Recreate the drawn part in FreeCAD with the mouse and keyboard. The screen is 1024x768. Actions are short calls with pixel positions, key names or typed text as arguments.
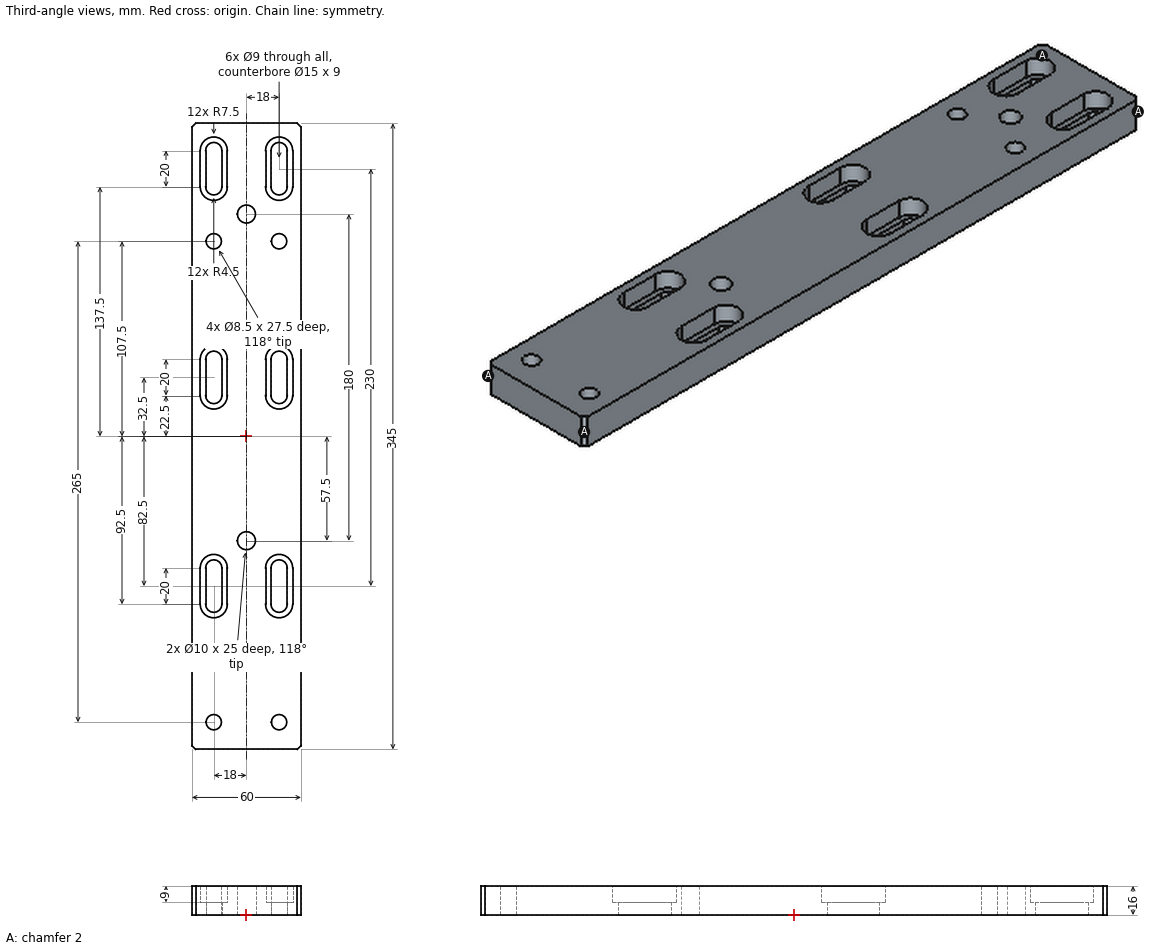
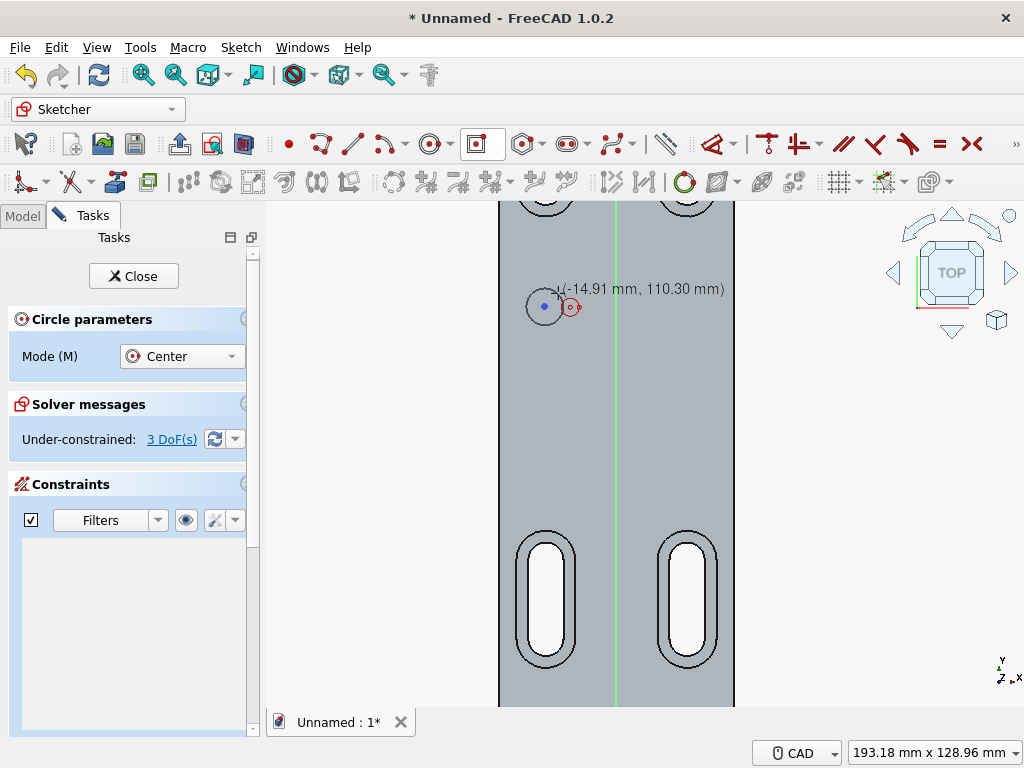
scroll(687, 305, up, 2)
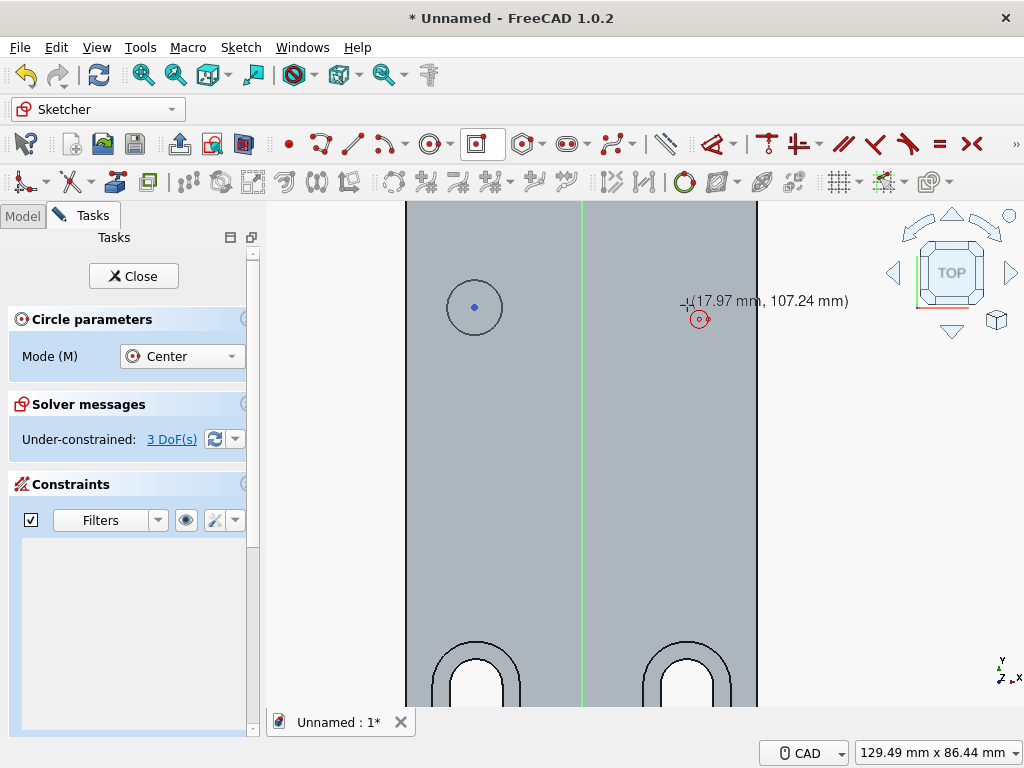
scroll(575, 296, down, 8)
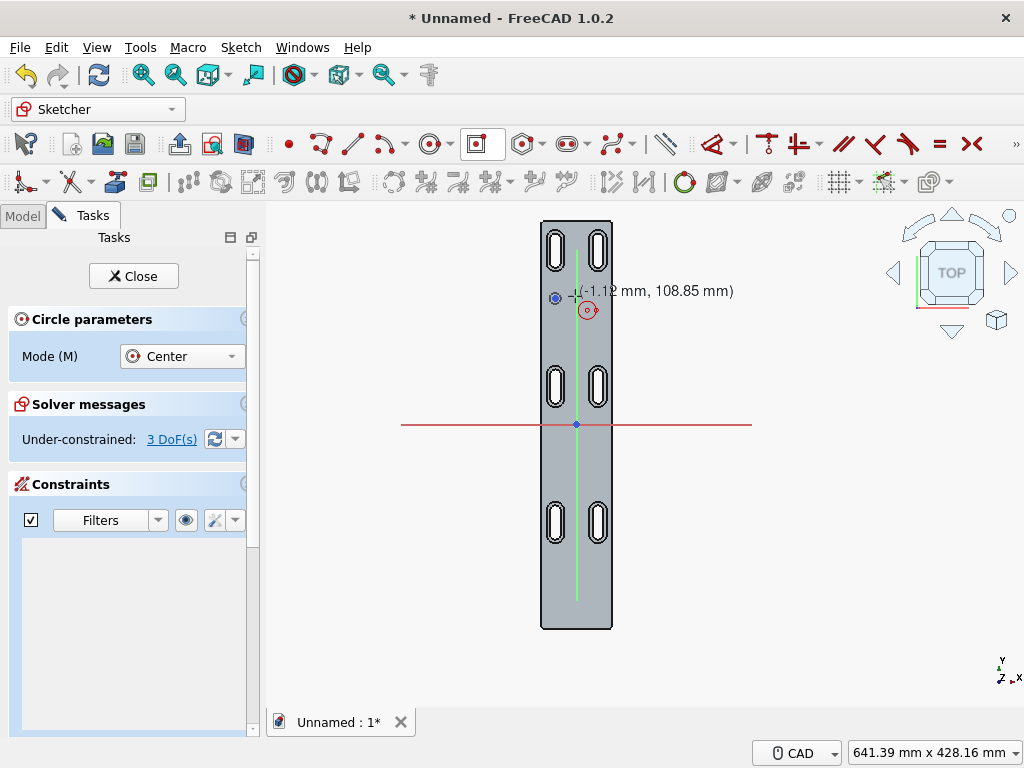
click(598, 298)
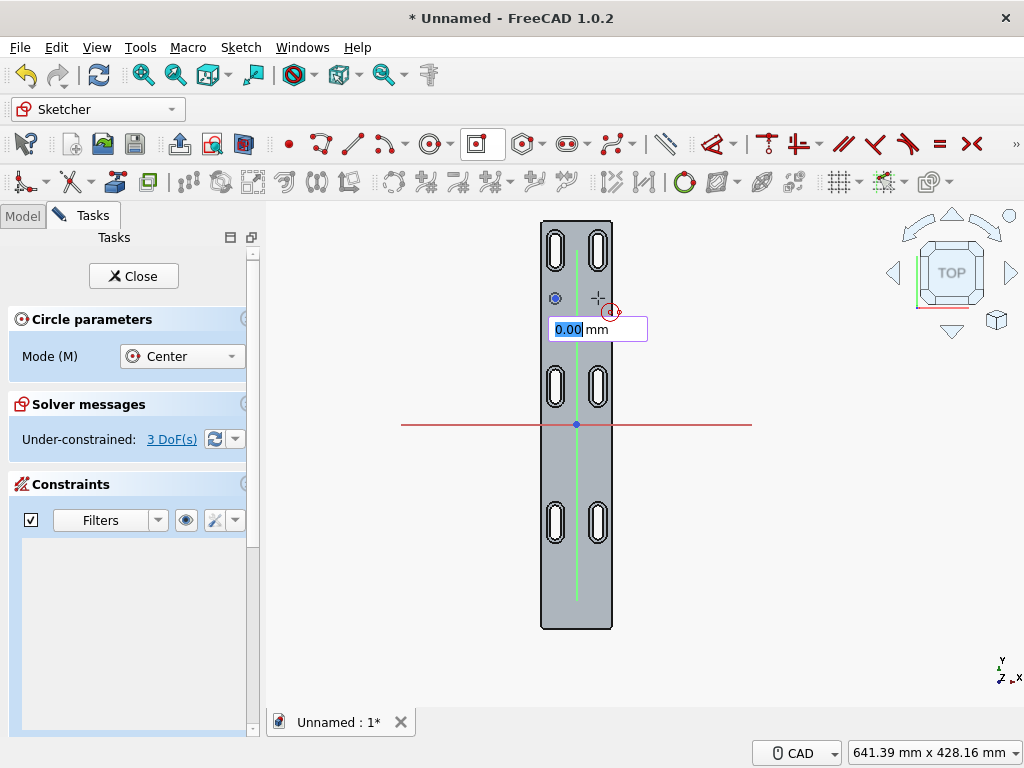
scroll(601, 294, up, 6)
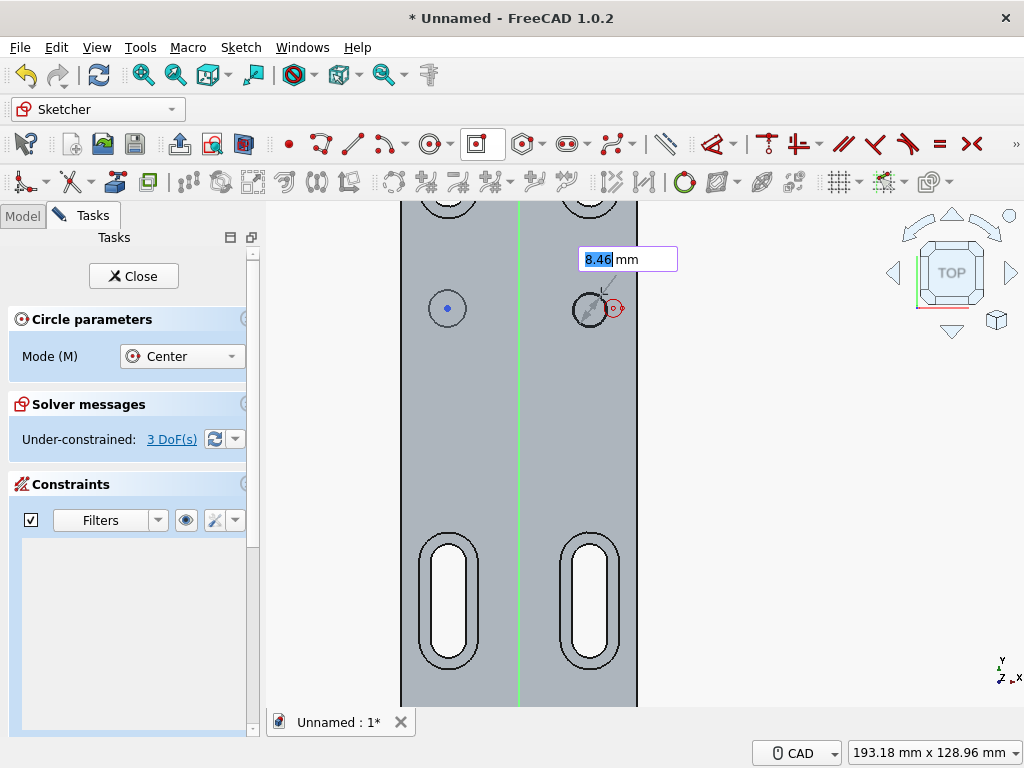
click(602, 295)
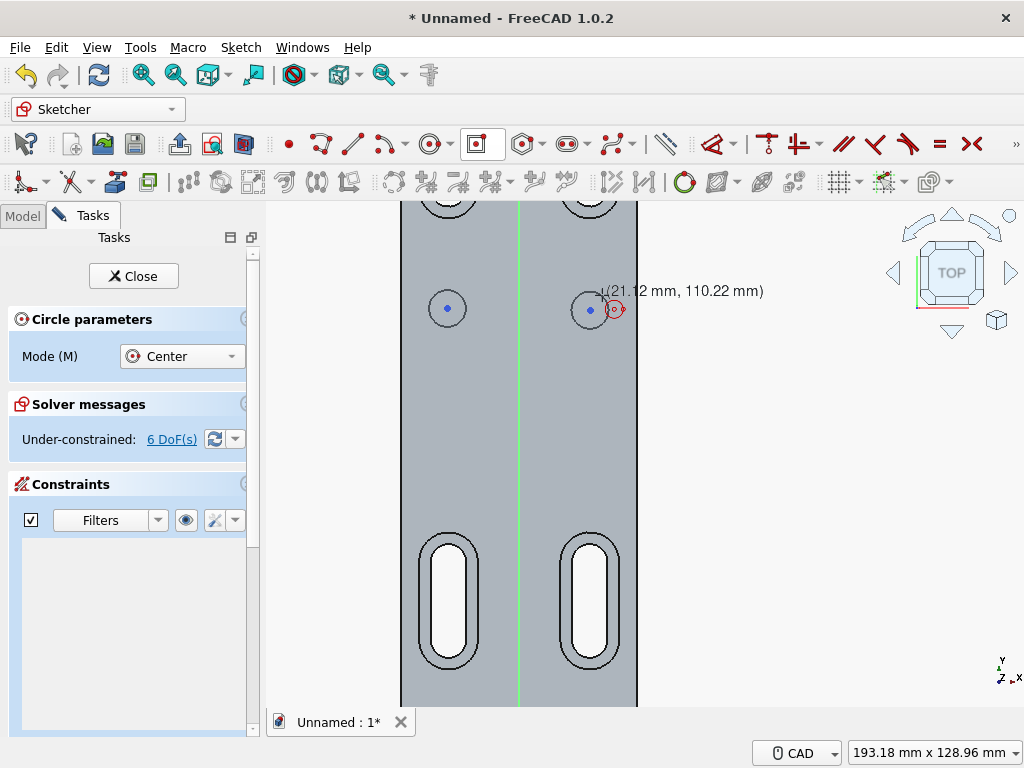
scroll(601, 293, down, 6)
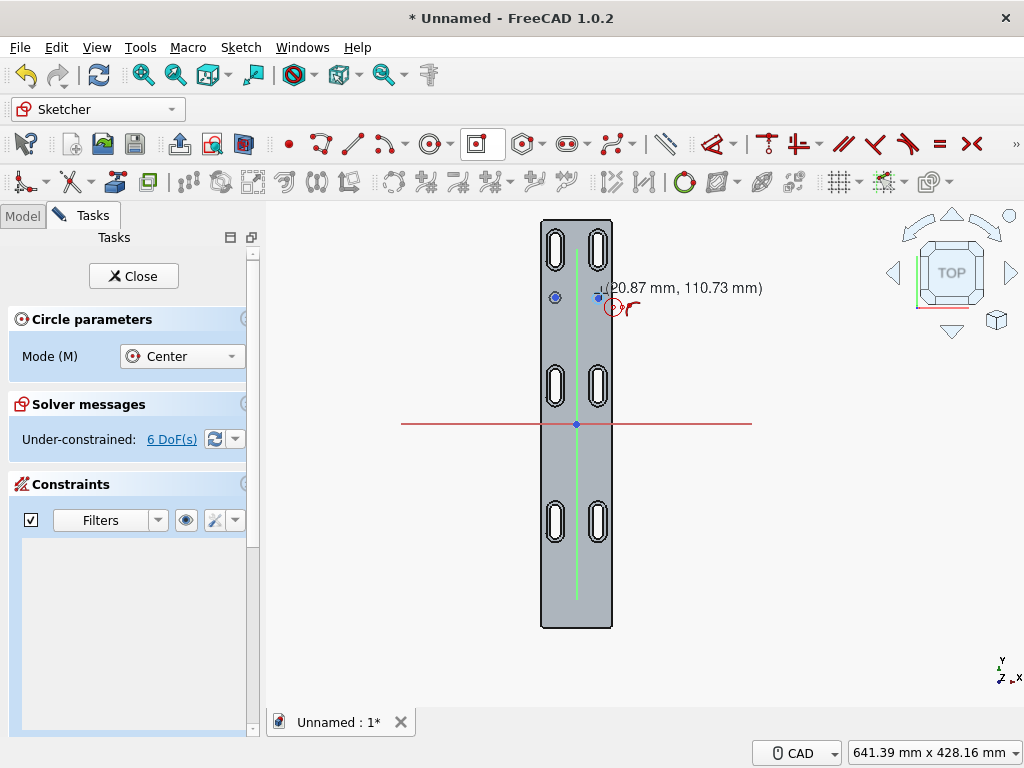
scroll(555, 610, up, 8)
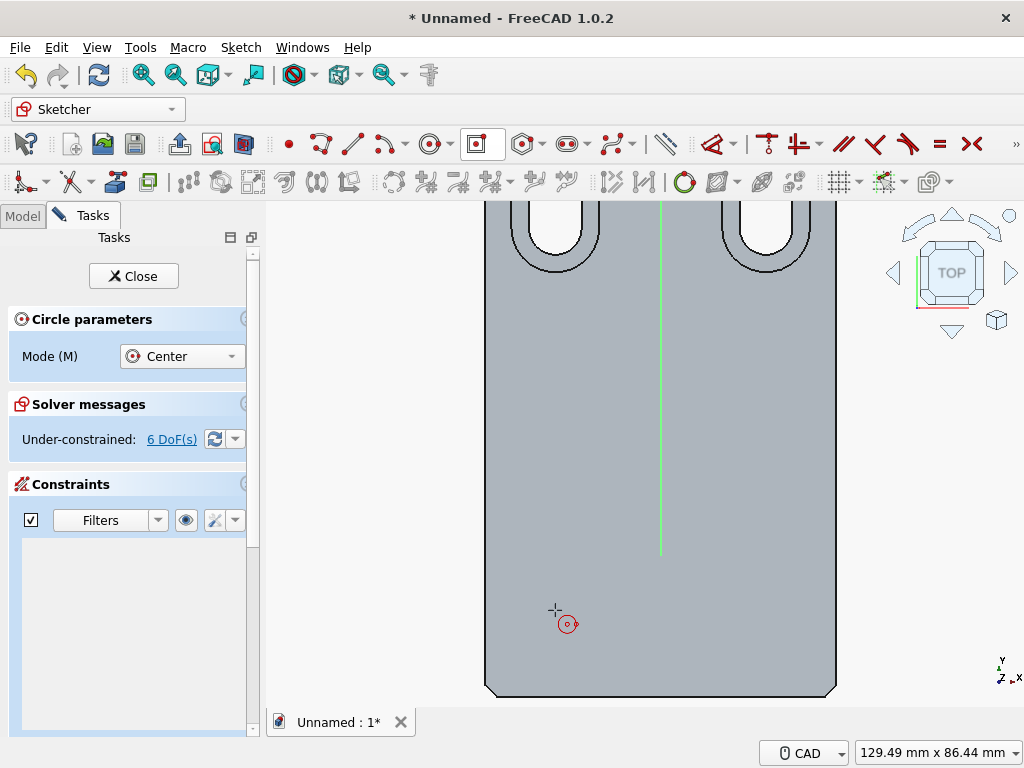
scroll(555, 611, down, 8)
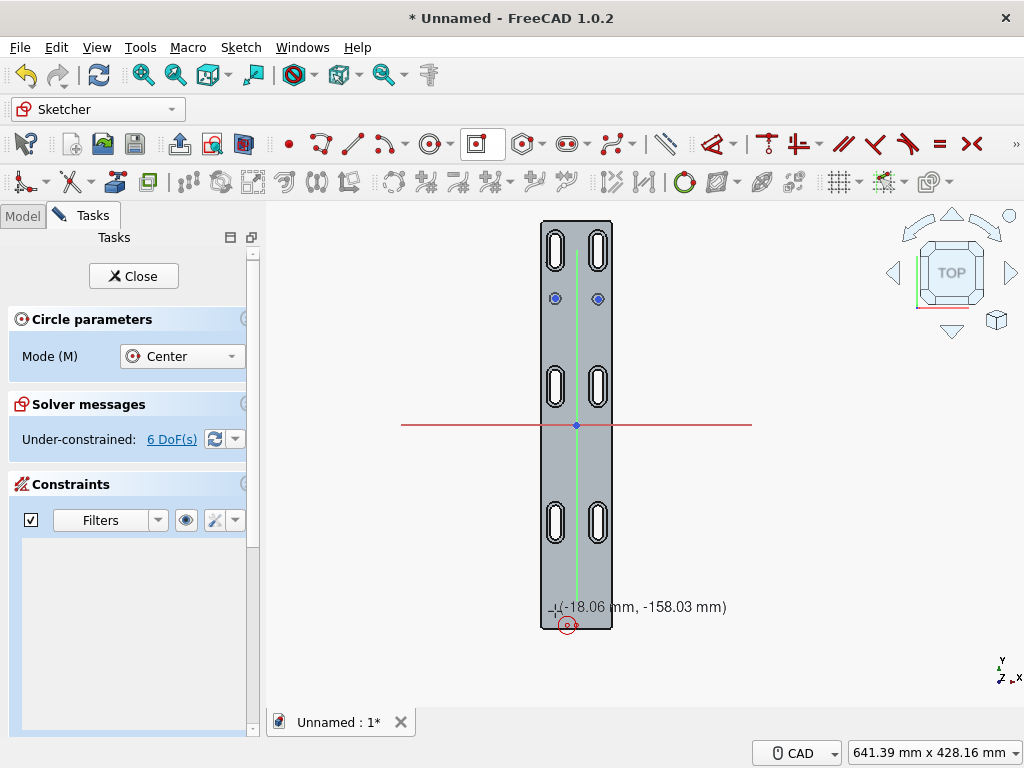
click(555, 611)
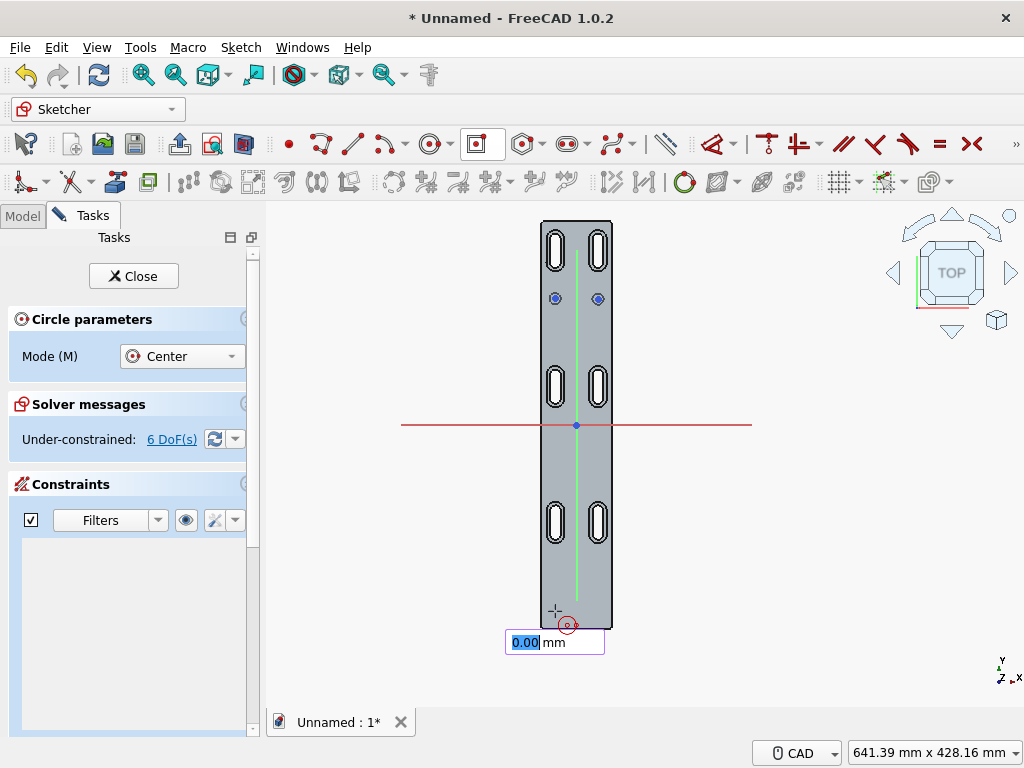
scroll(559, 608, up, 6)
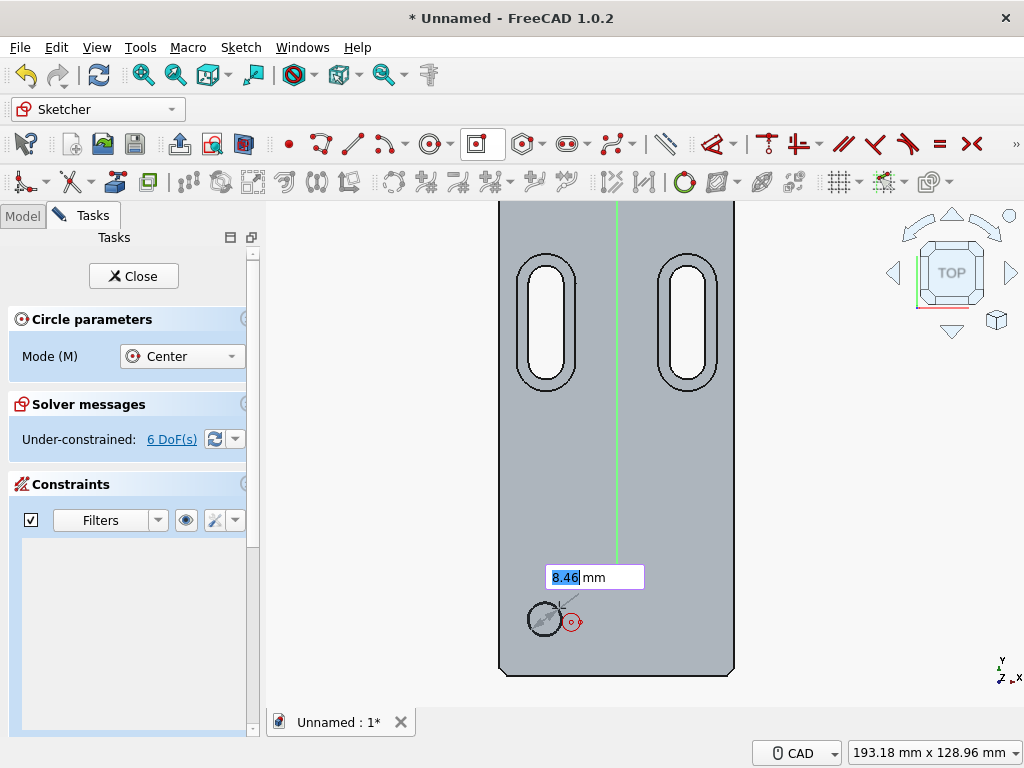
click(558, 605)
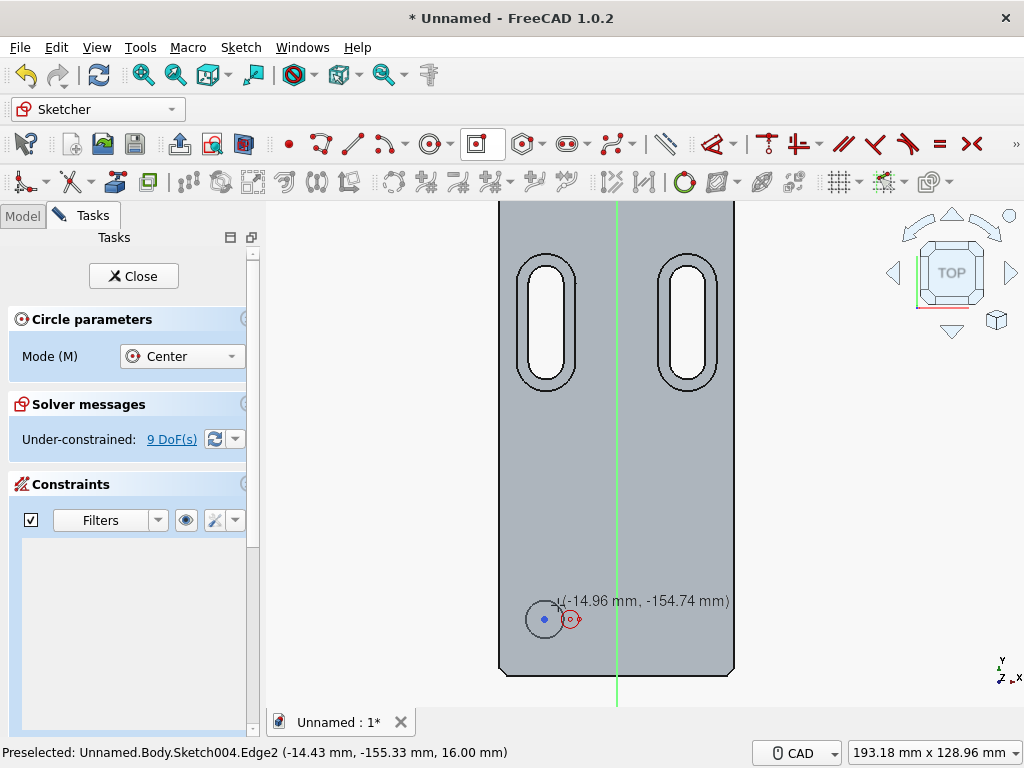
scroll(687, 617, up, 2)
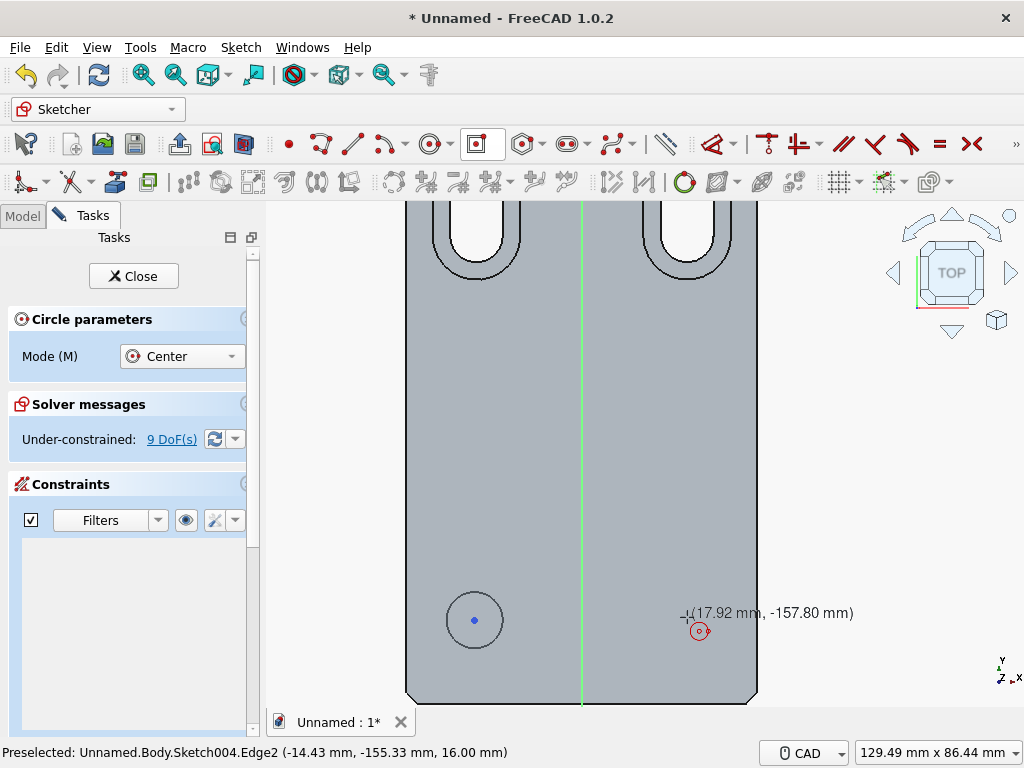
scroll(575, 609, down, 8)